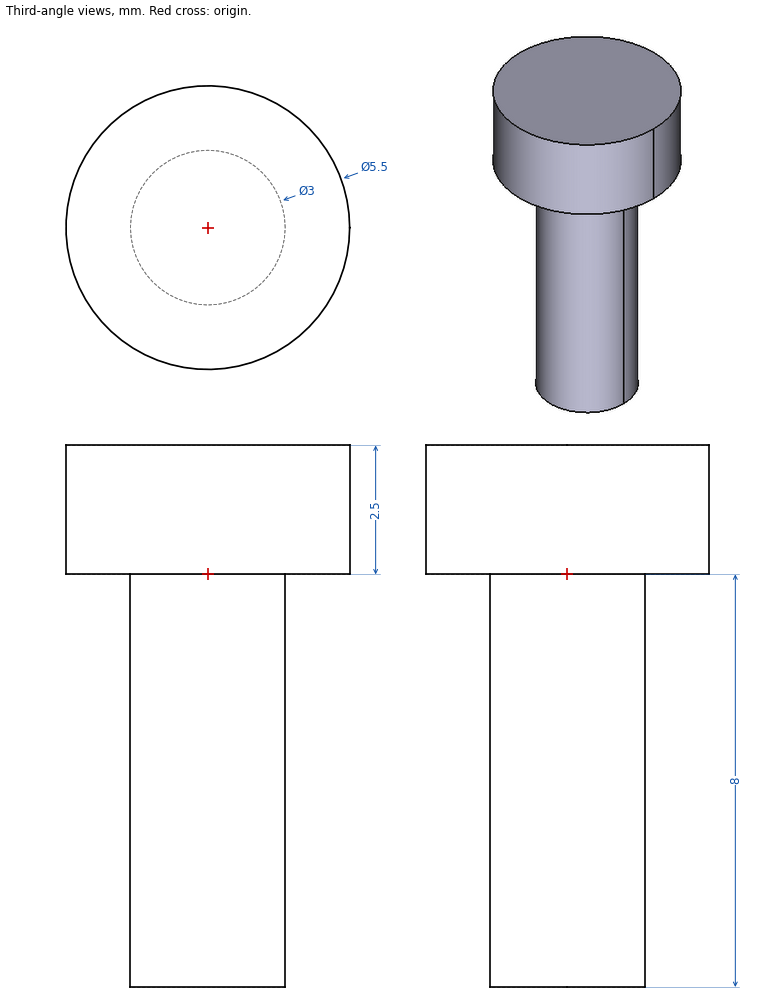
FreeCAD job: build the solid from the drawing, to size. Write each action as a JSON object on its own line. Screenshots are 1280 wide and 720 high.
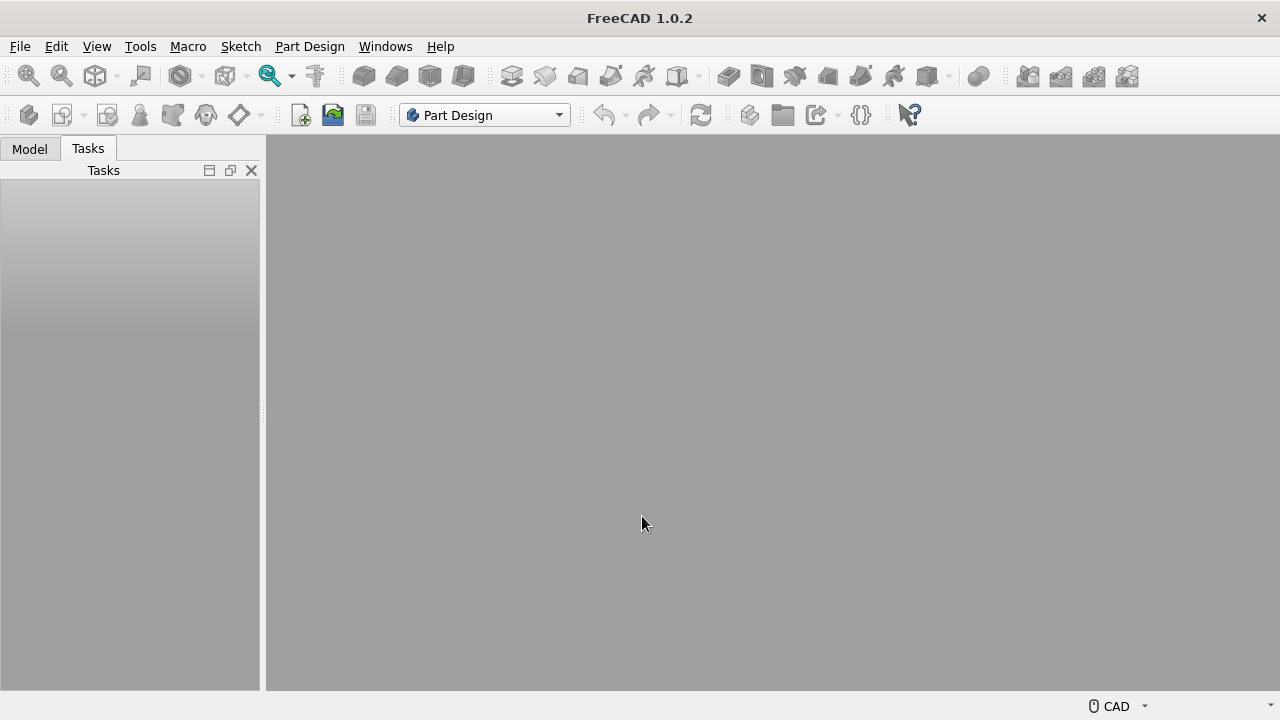
{"action": "left_click", "coordinate": [300, 116]}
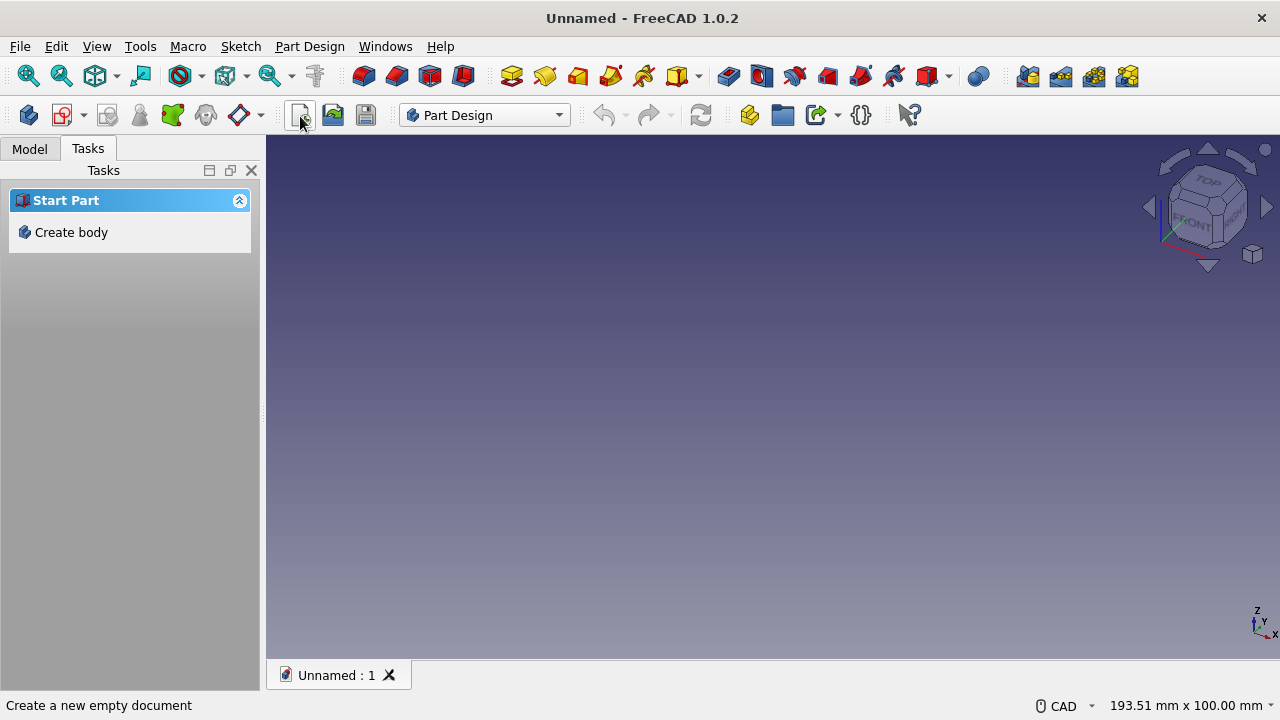
{"action": "left_click", "coordinate": [62, 116]}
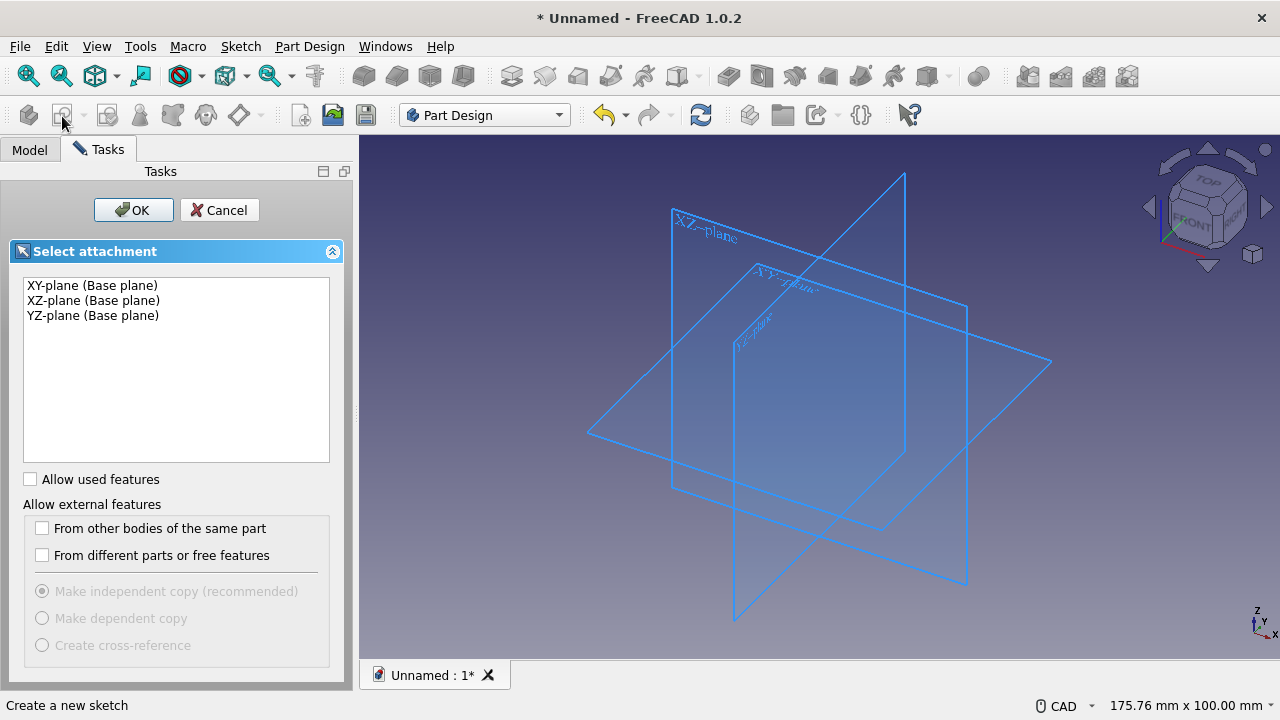
{"action": "left_click", "coordinate": [84, 286]}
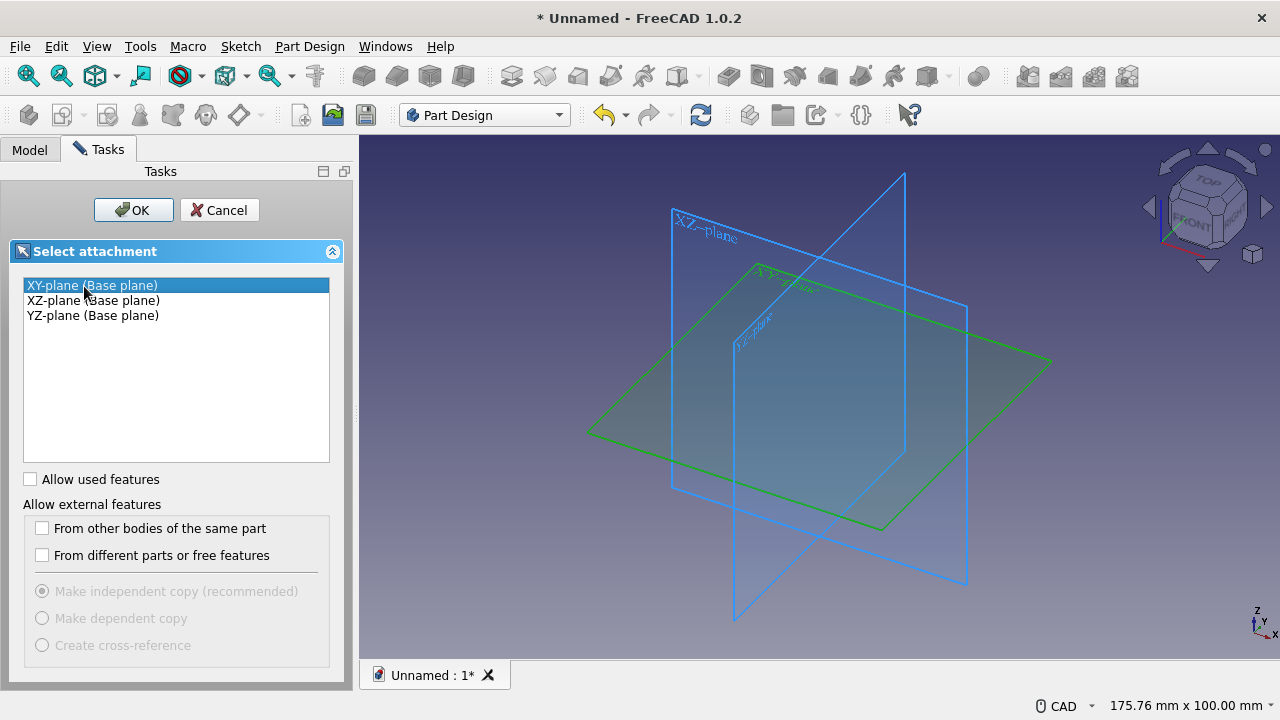
{"action": "left_click", "coordinate": [134, 210]}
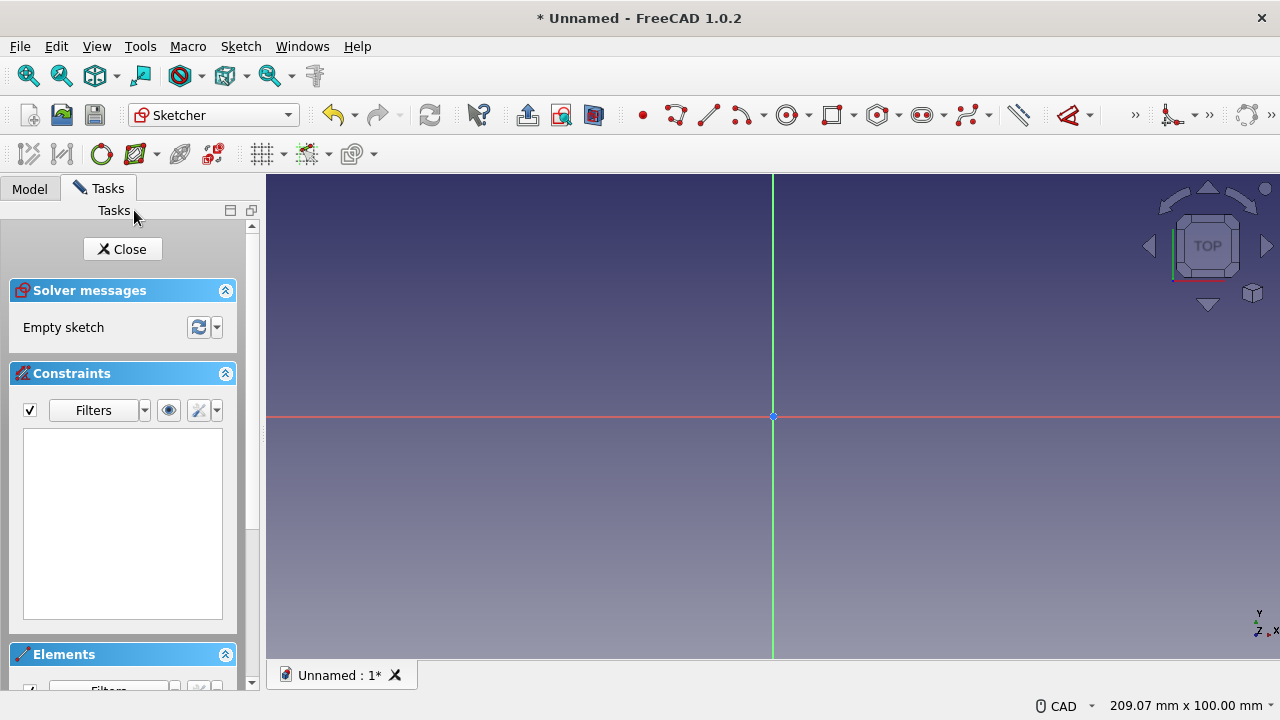
{"action": "scroll", "coordinate": [777, 416], "scroll_direction": "up", "scroll_amount": 15}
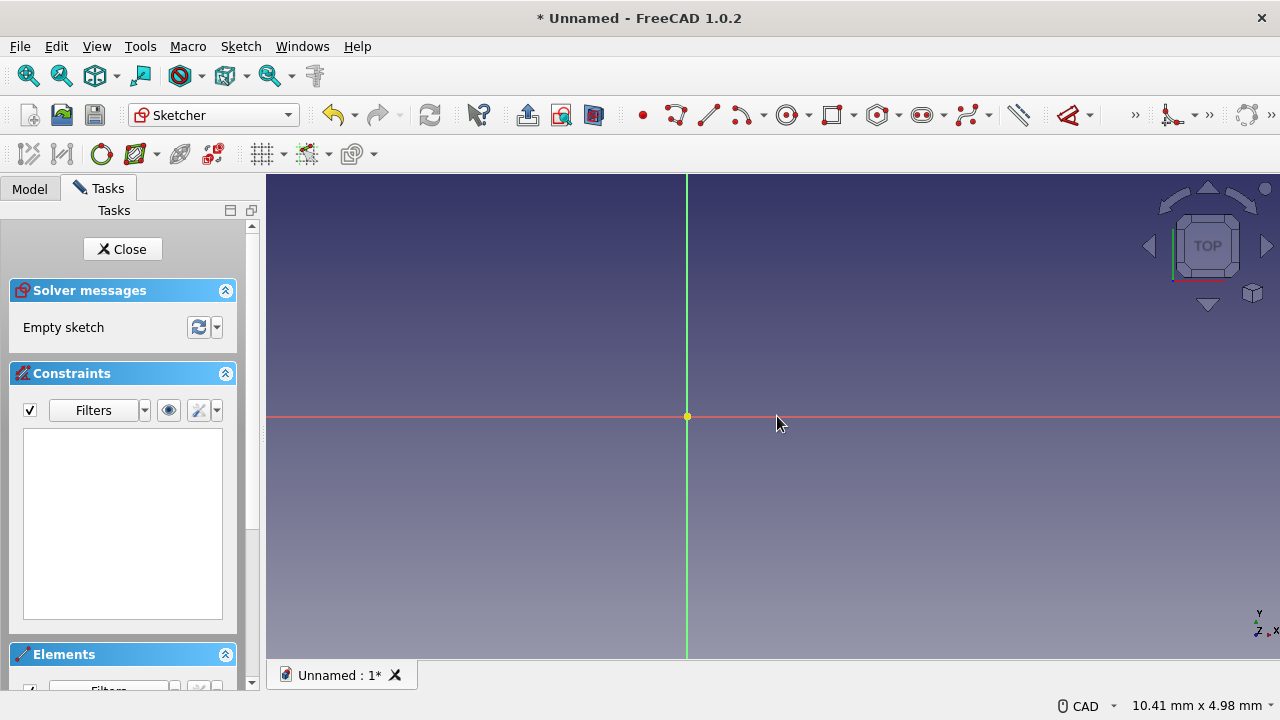
{"action": "left_click", "coordinate": [786, 116]}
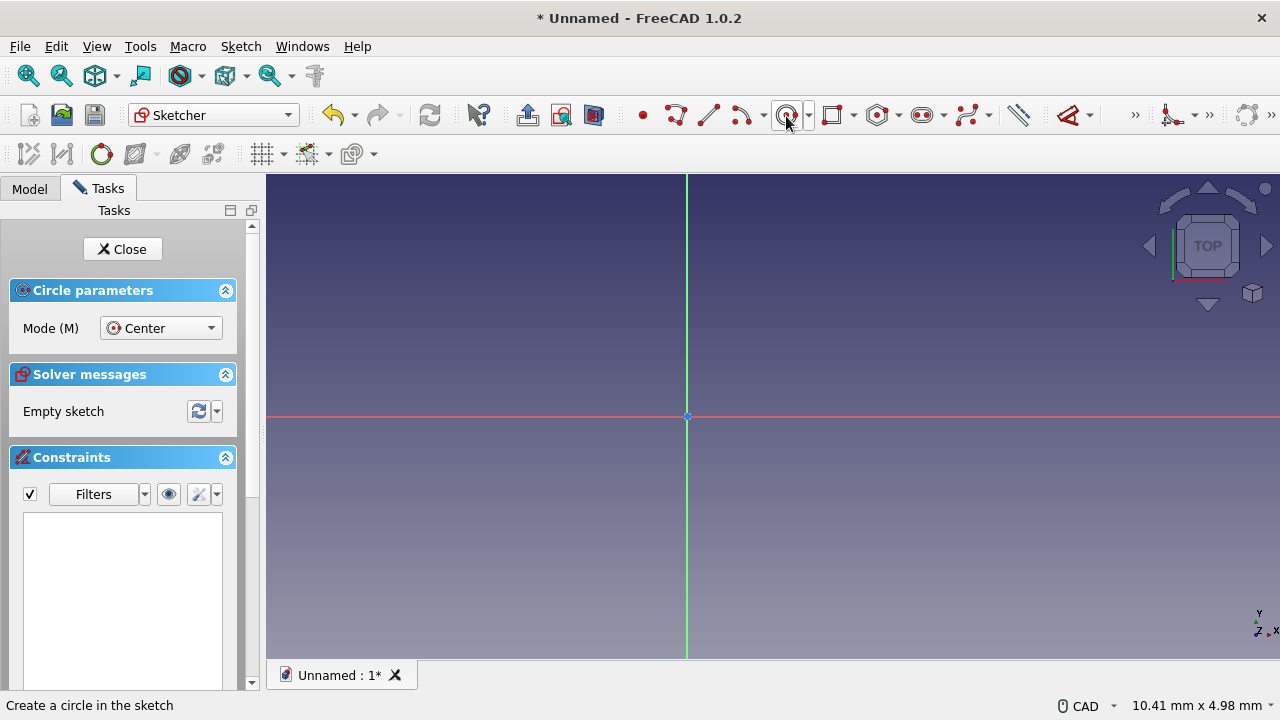
{"action": "left_click", "coordinate": [687, 416]}
{"action": "left_click", "coordinate": [790, 313]}
{"action": "key", "text": "Escape"}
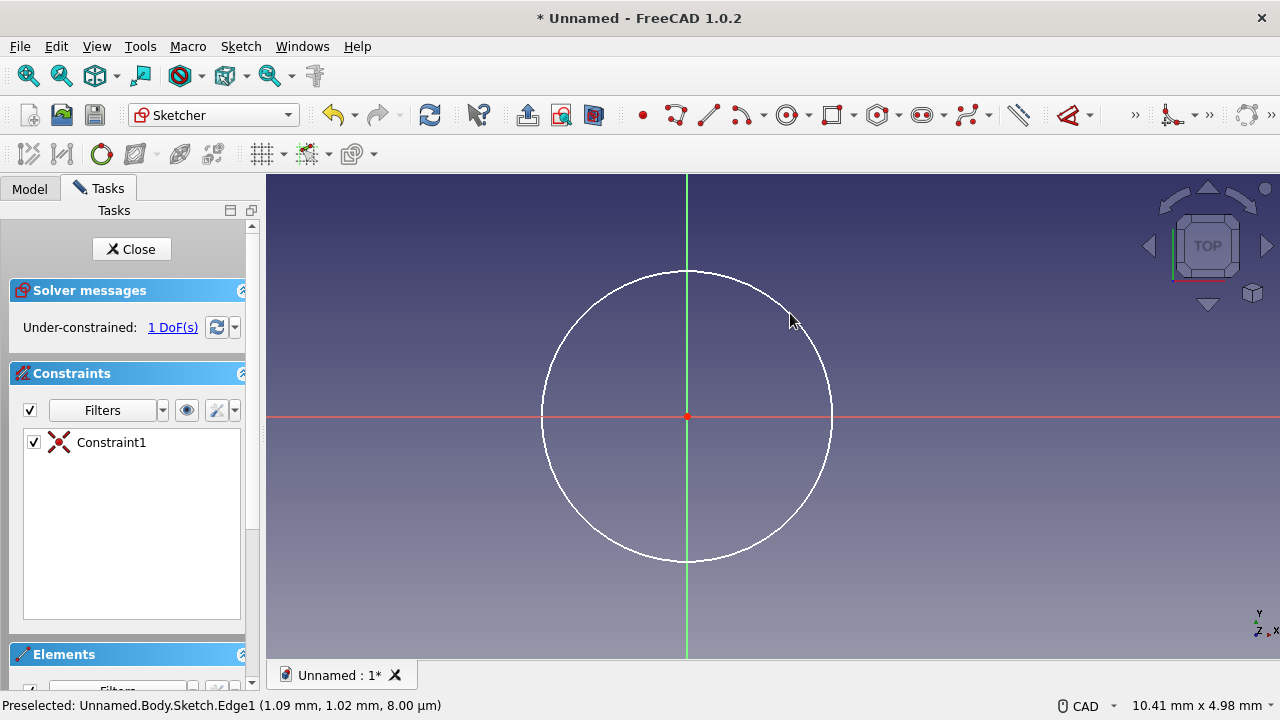
{"action": "left_click", "coordinate": [789, 313]}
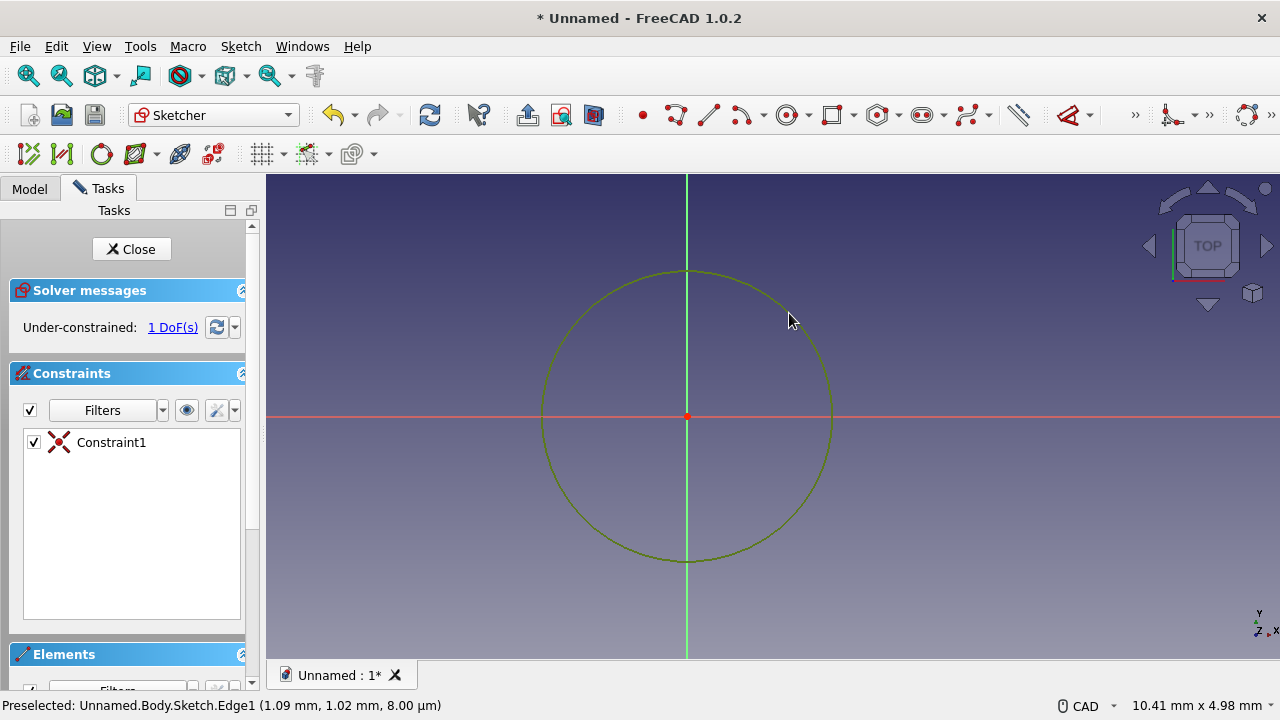
{"action": "key", "text": "k o"}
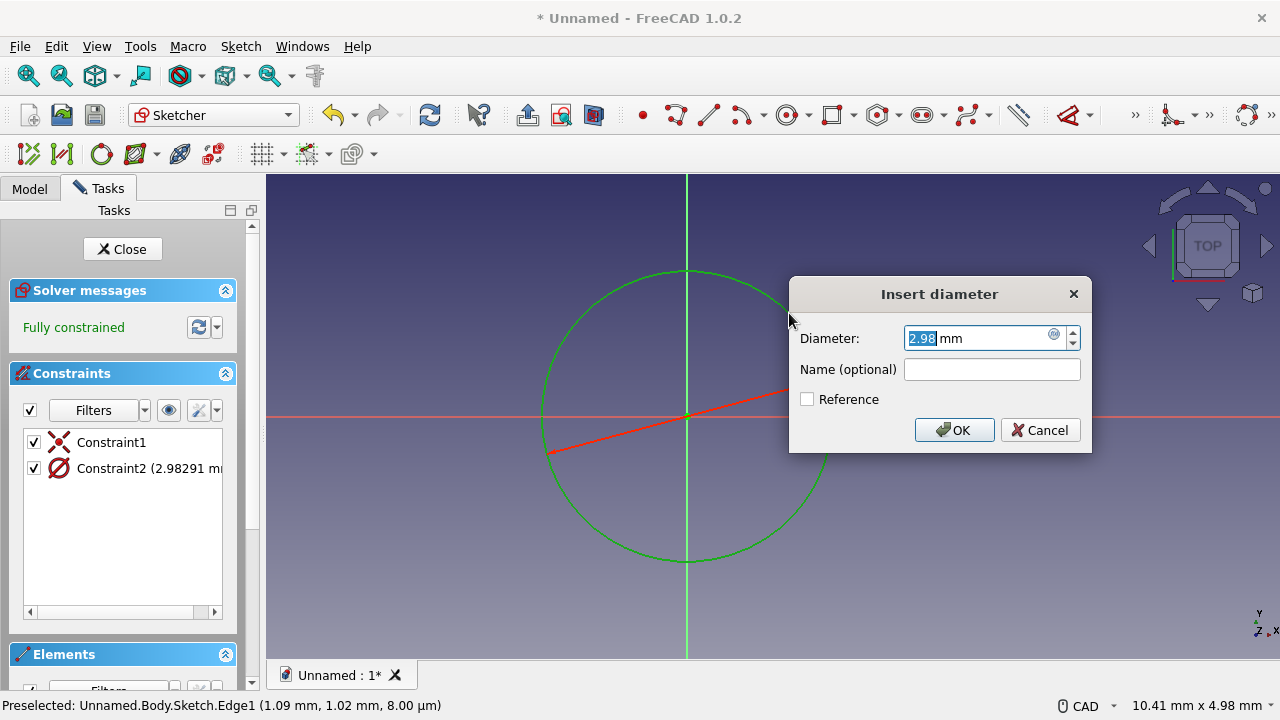
{"action": "type", "text": "3"}
{"action": "key", "text": "Return"}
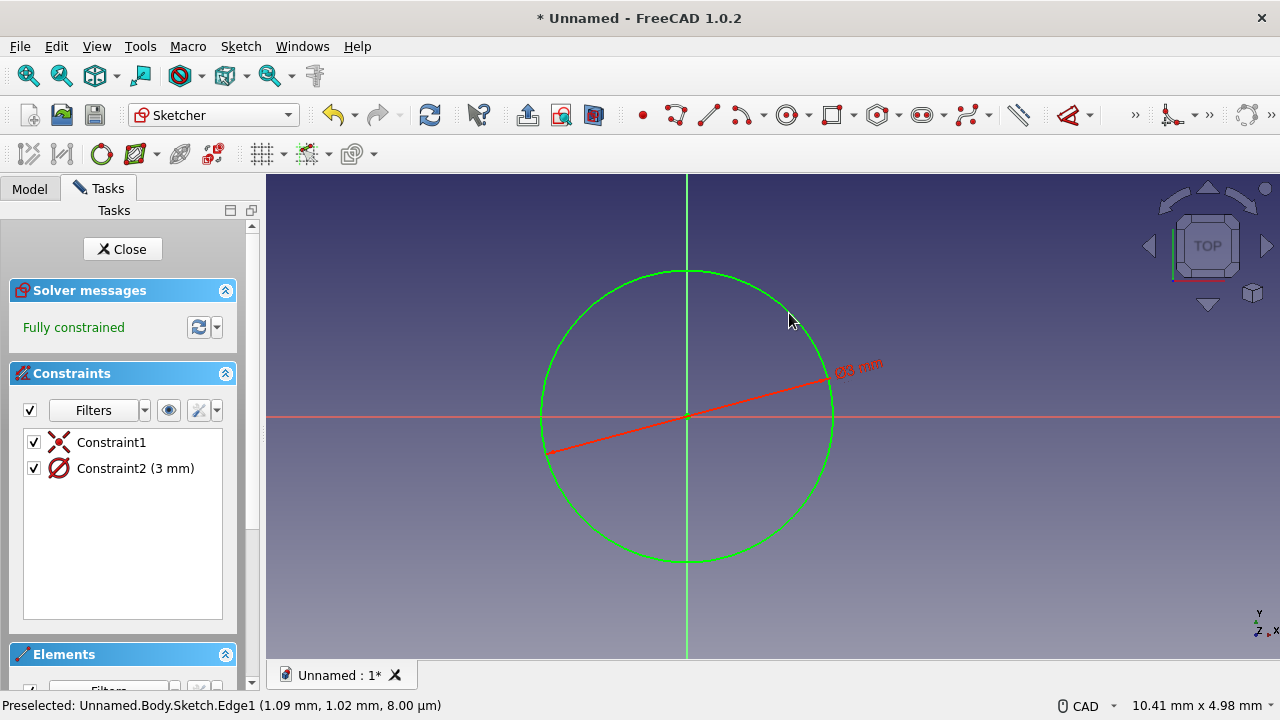
{"action": "left_click", "coordinate": [123, 249]}